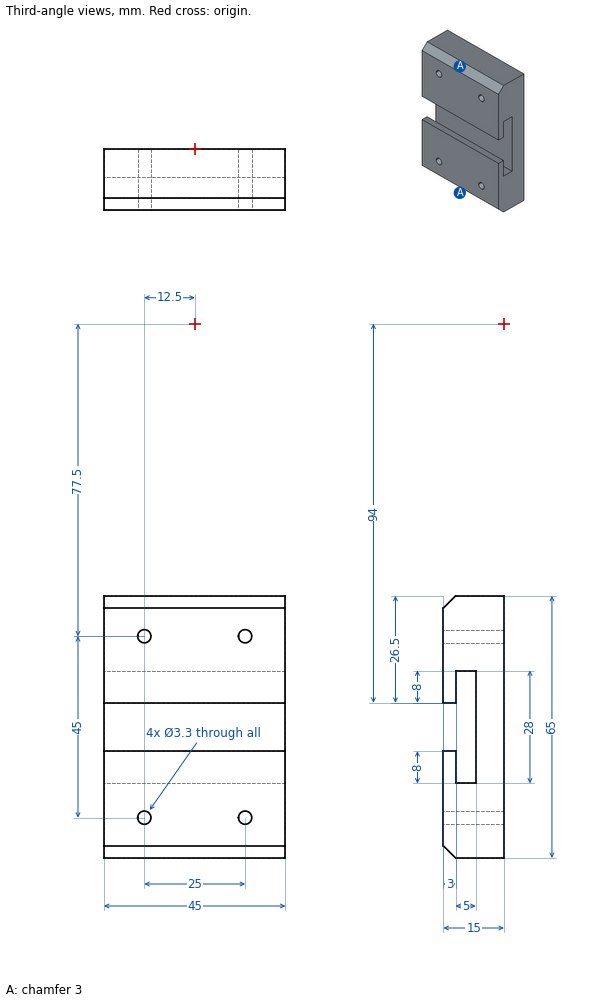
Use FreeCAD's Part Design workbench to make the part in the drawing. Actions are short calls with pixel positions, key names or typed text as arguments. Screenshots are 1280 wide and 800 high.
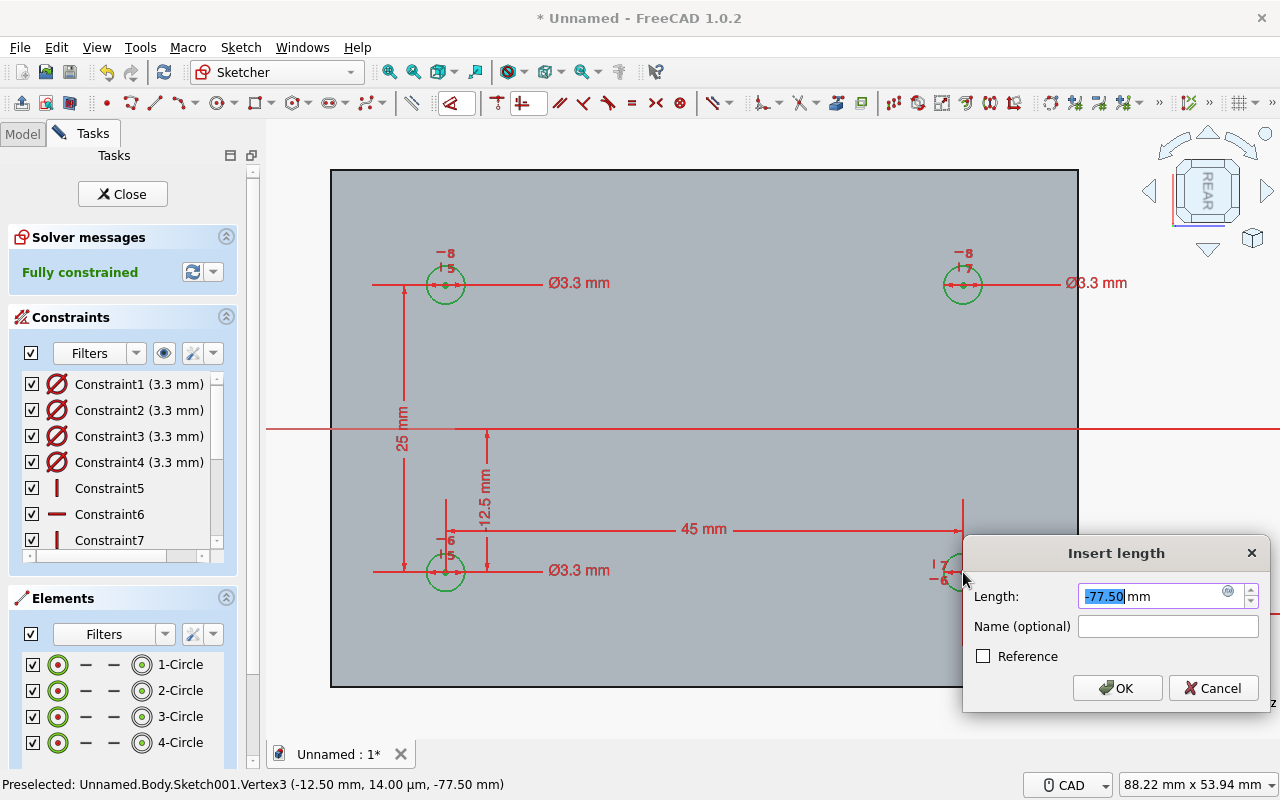
text(-77.5)
key(Return)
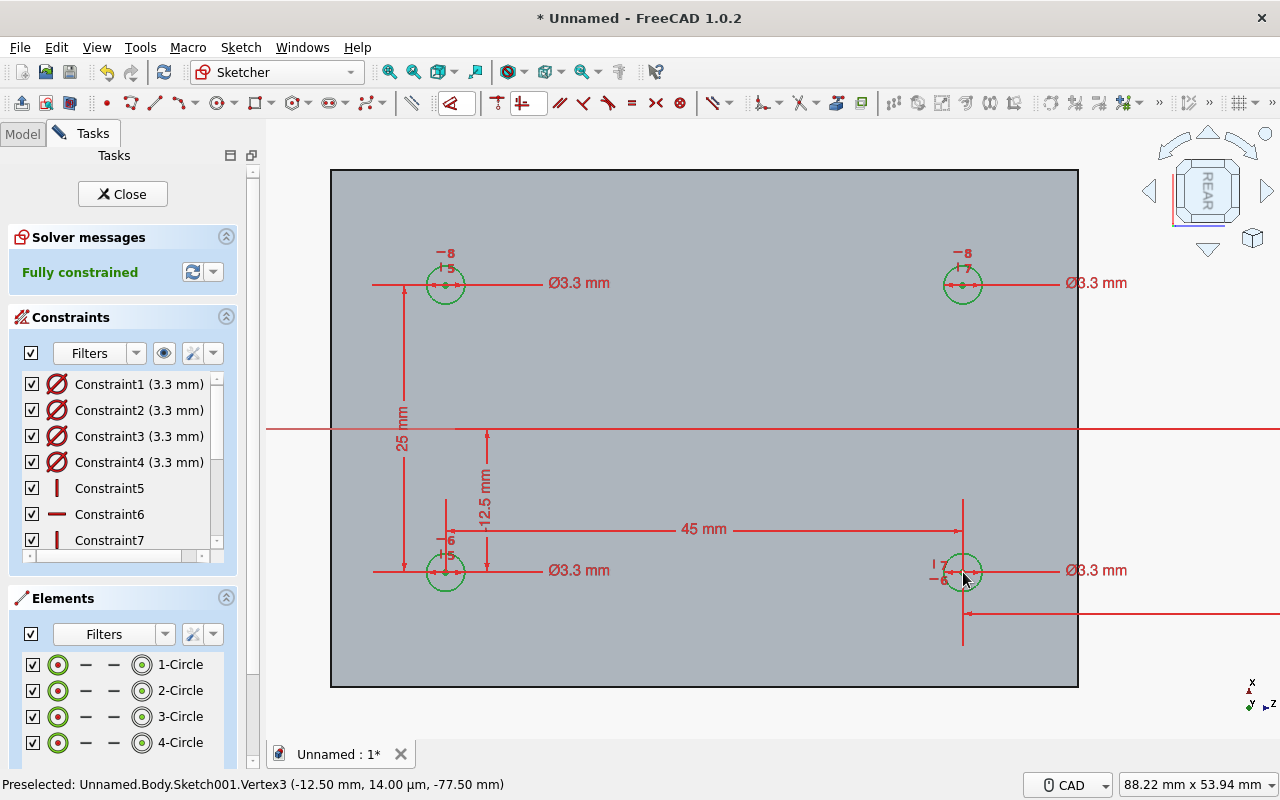
click(123, 194)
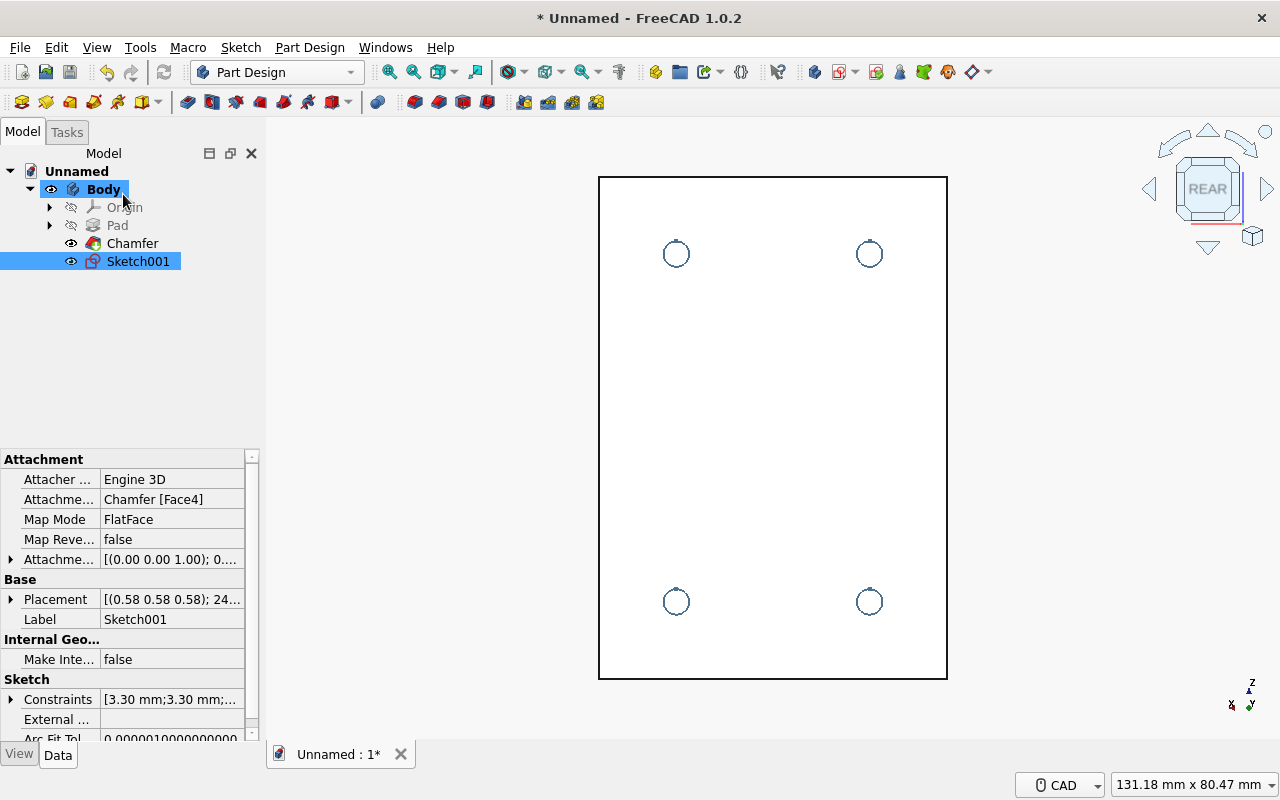
click(212, 102)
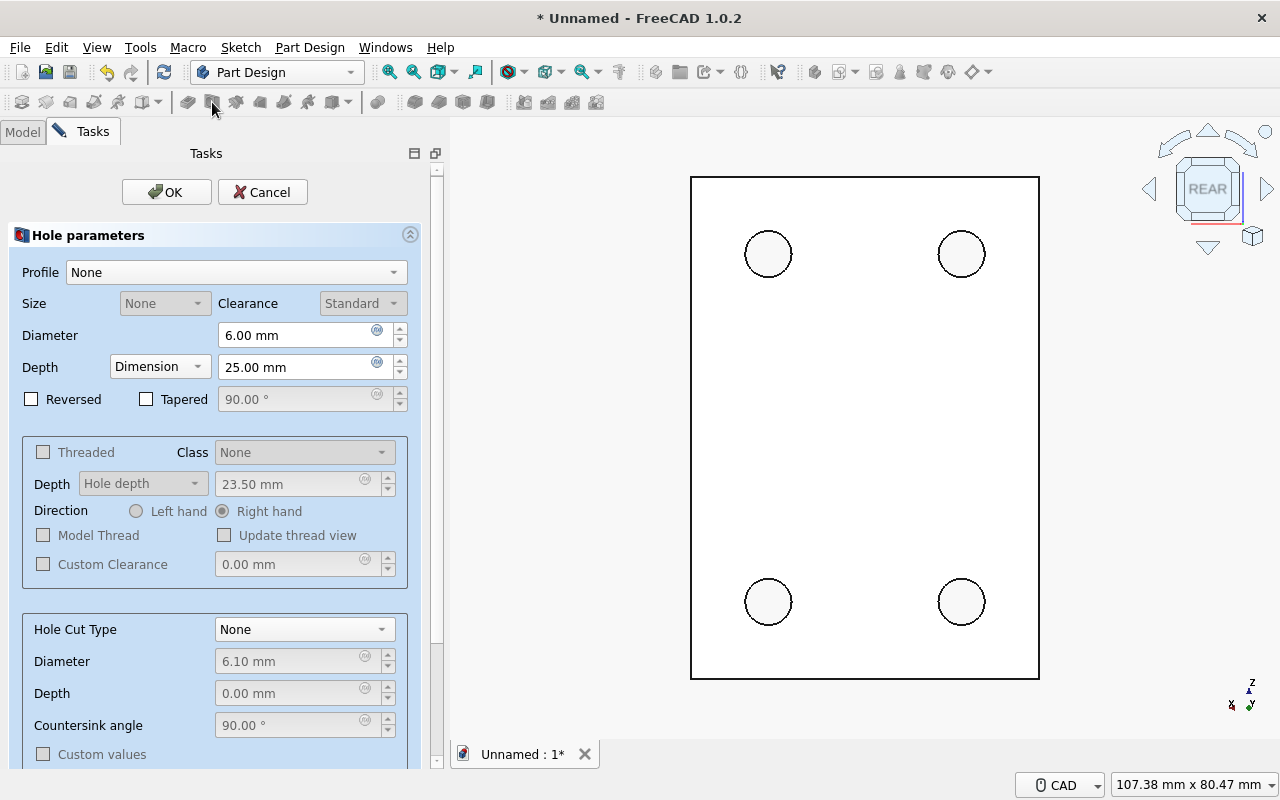
triple_click(305, 335)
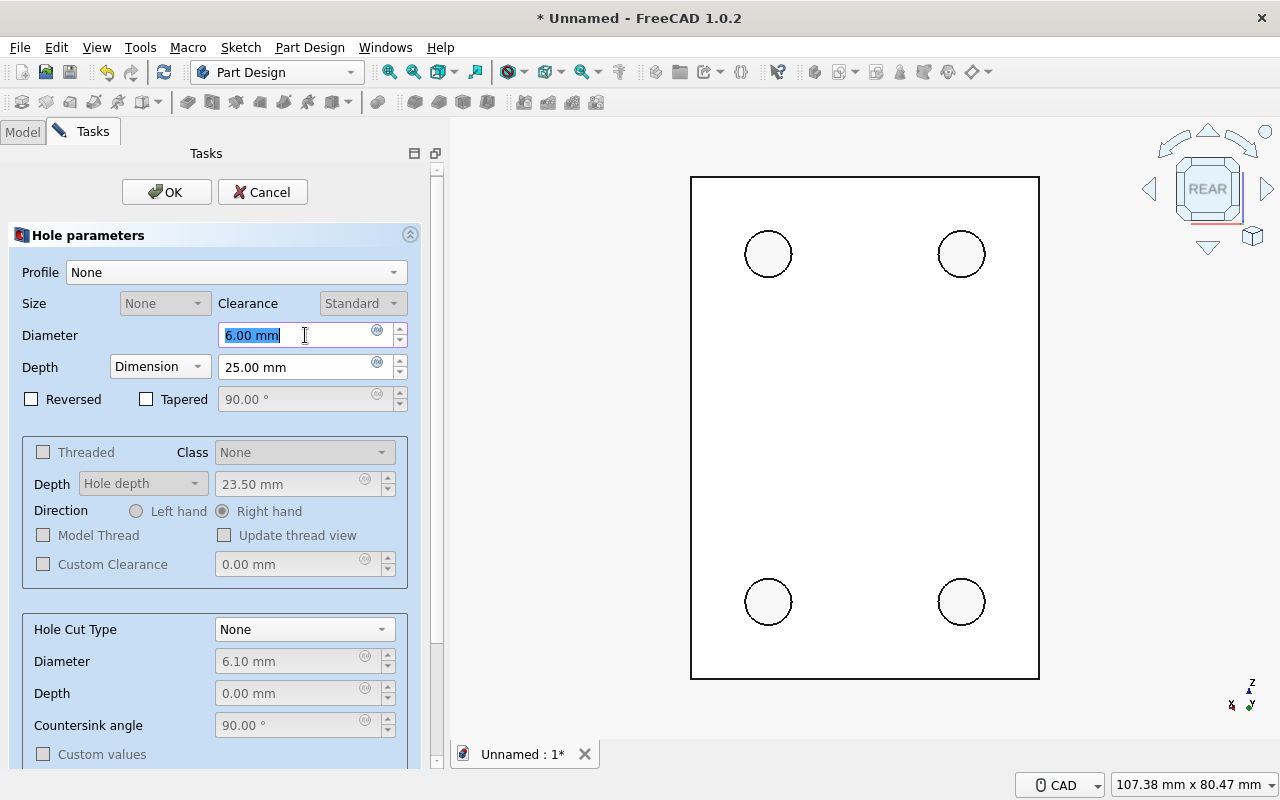
text(3.3)
key(Tab)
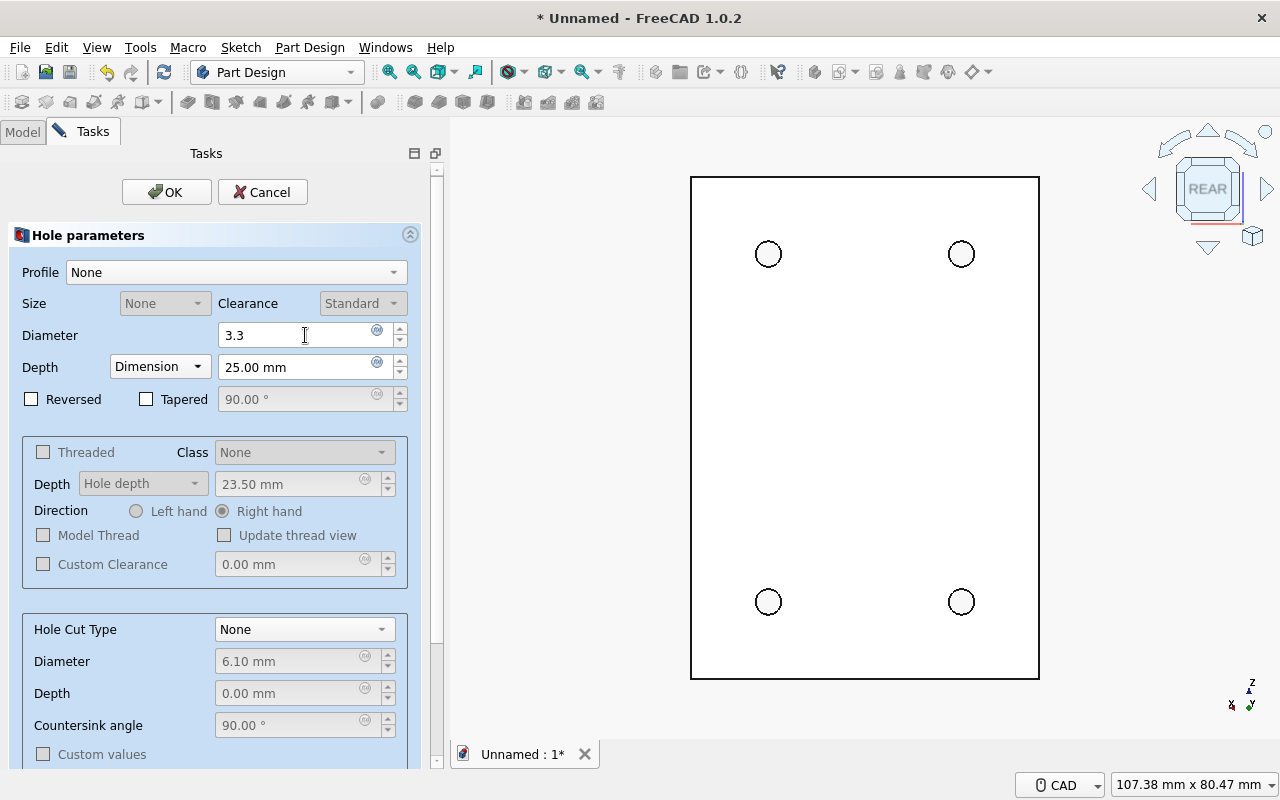
click(161, 366)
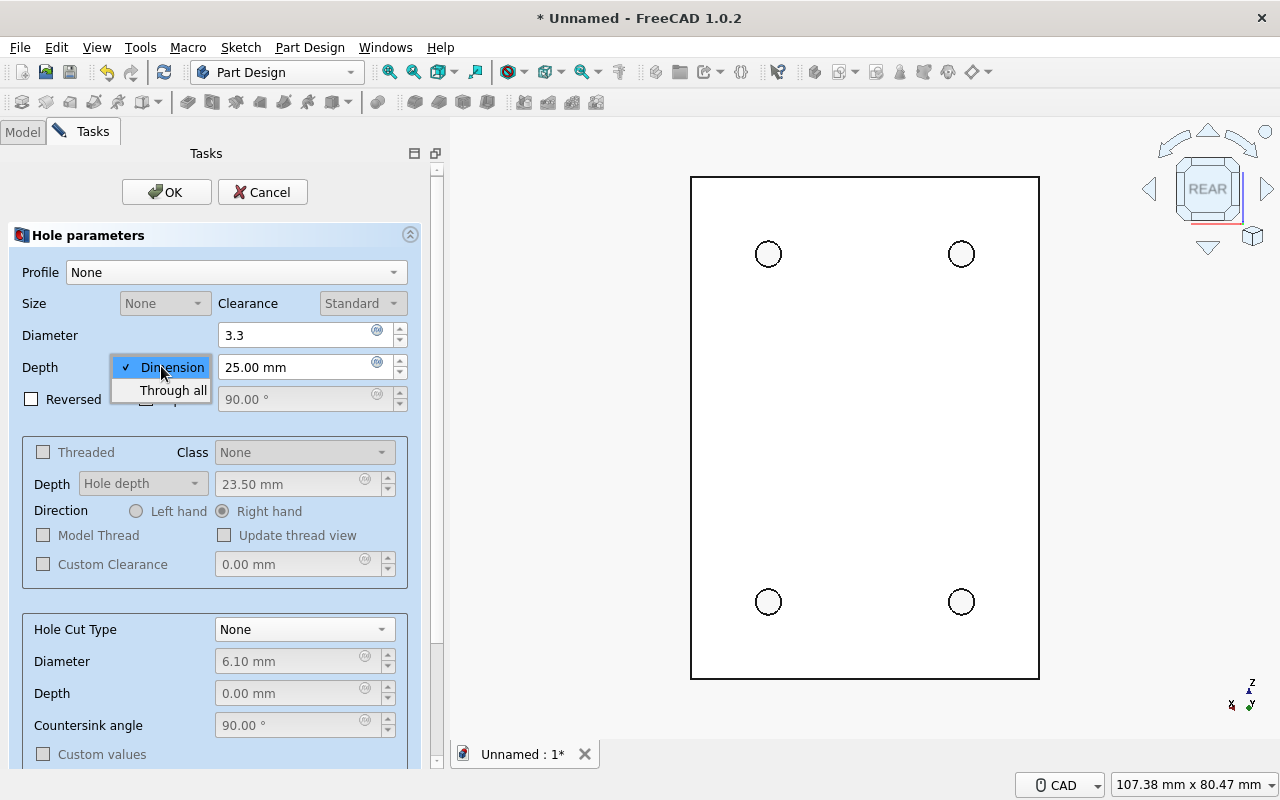
click(160, 390)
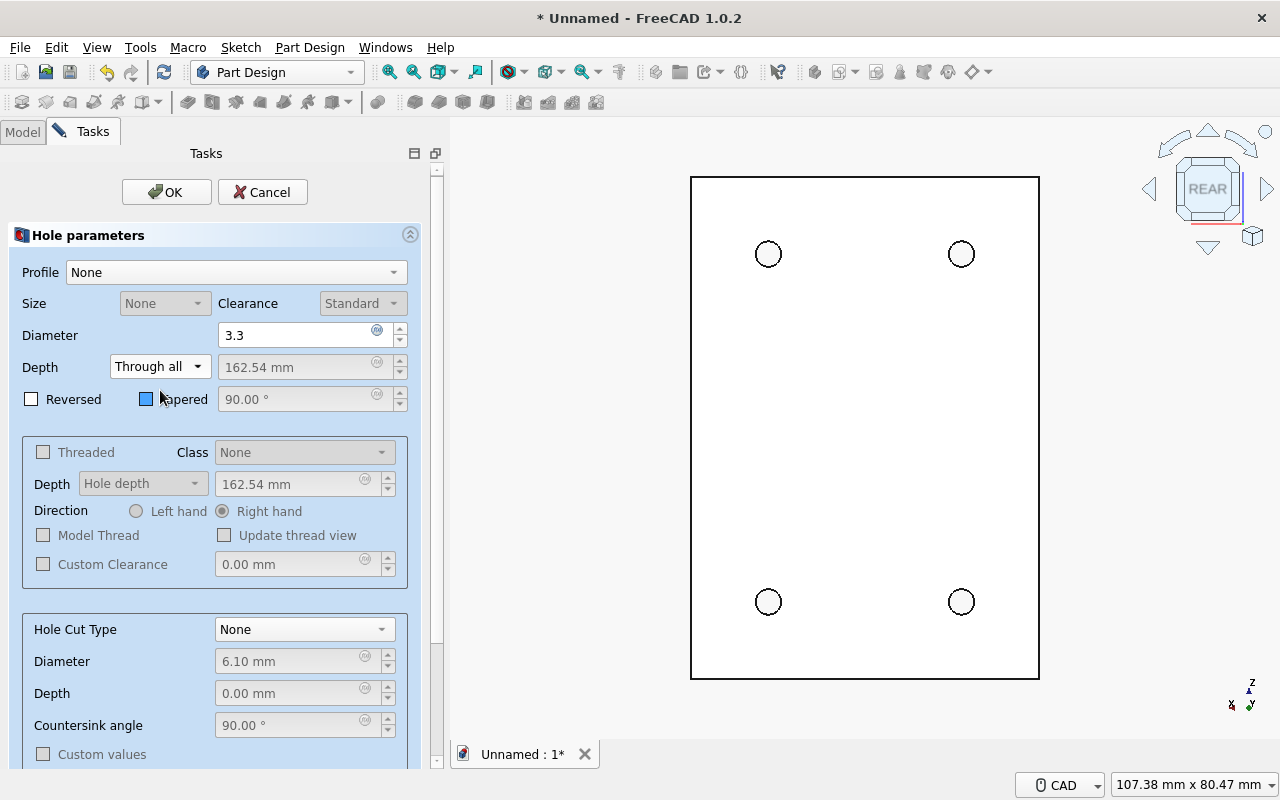
click(167, 192)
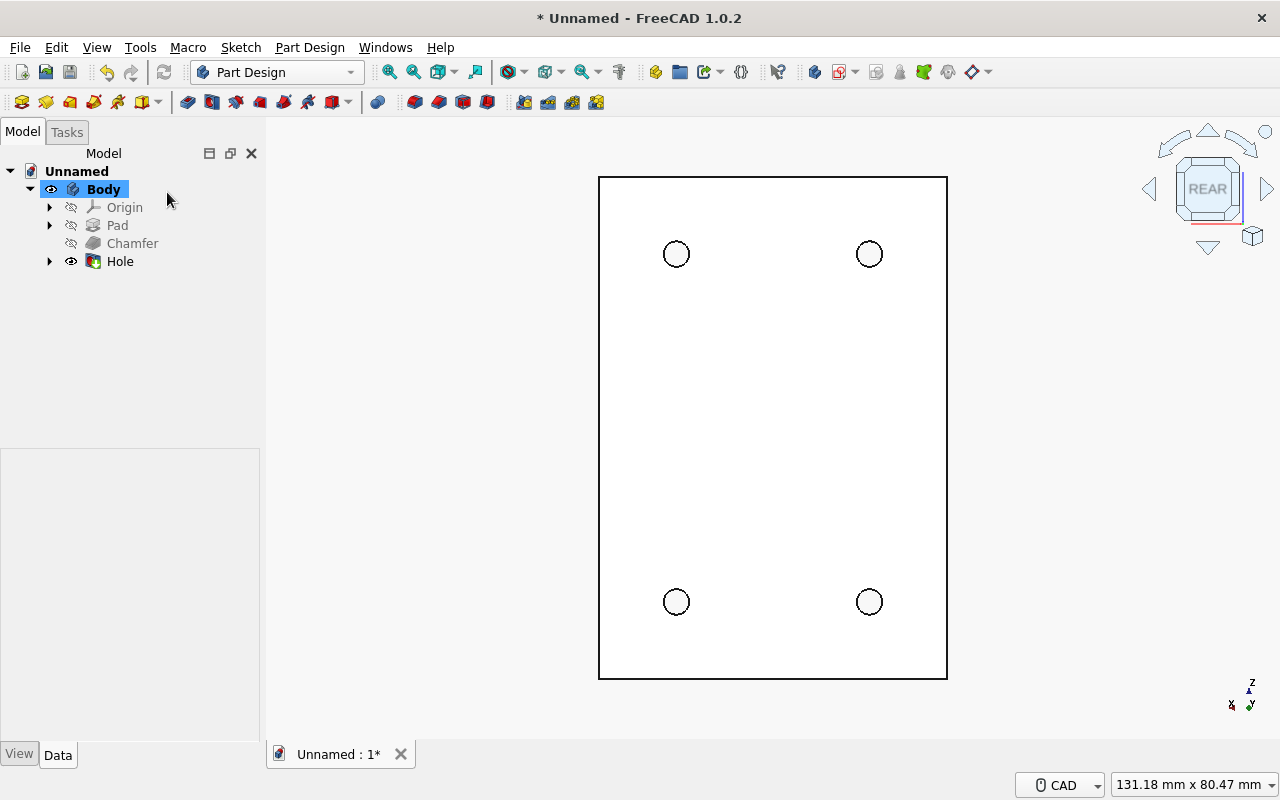
key(0)